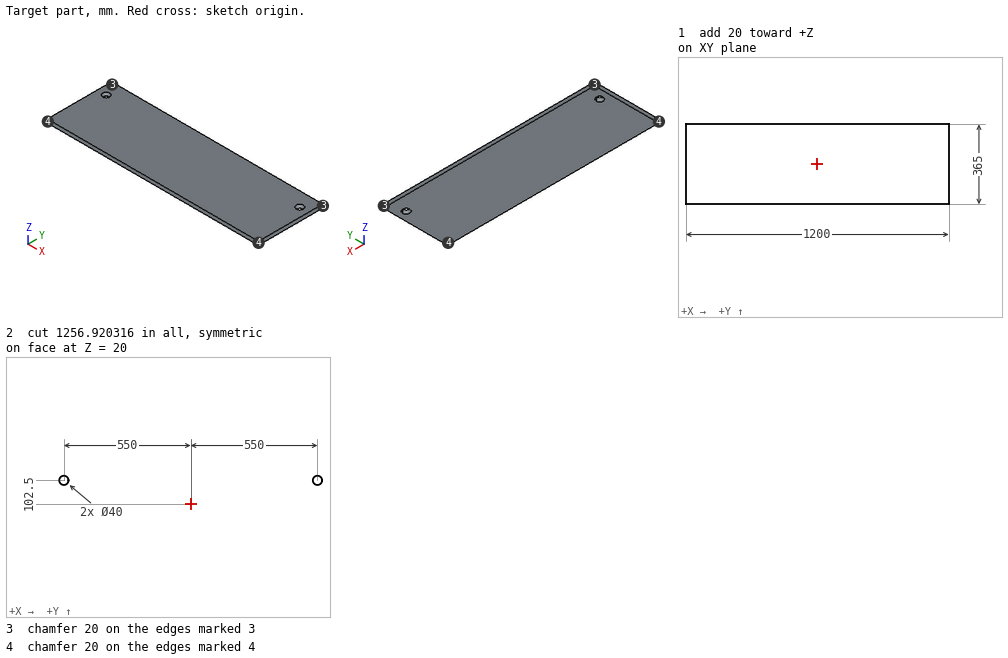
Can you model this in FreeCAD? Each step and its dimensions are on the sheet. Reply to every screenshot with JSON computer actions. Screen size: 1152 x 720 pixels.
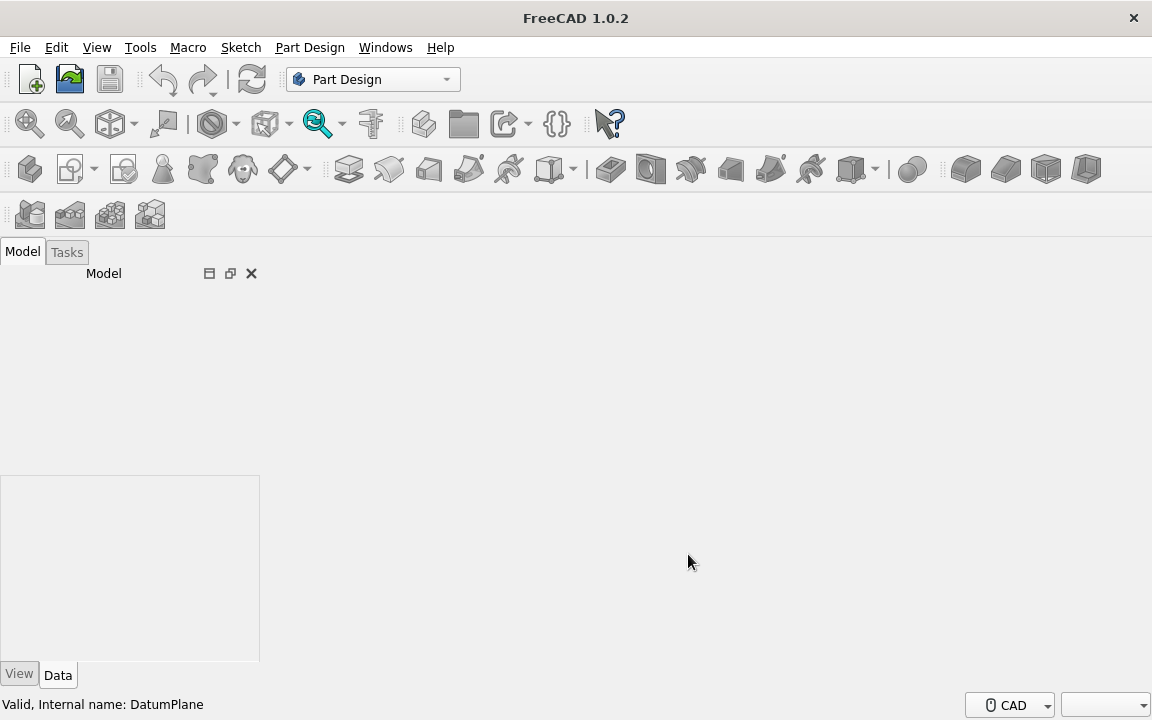
{"action": "left_click", "coordinate": [30, 80]}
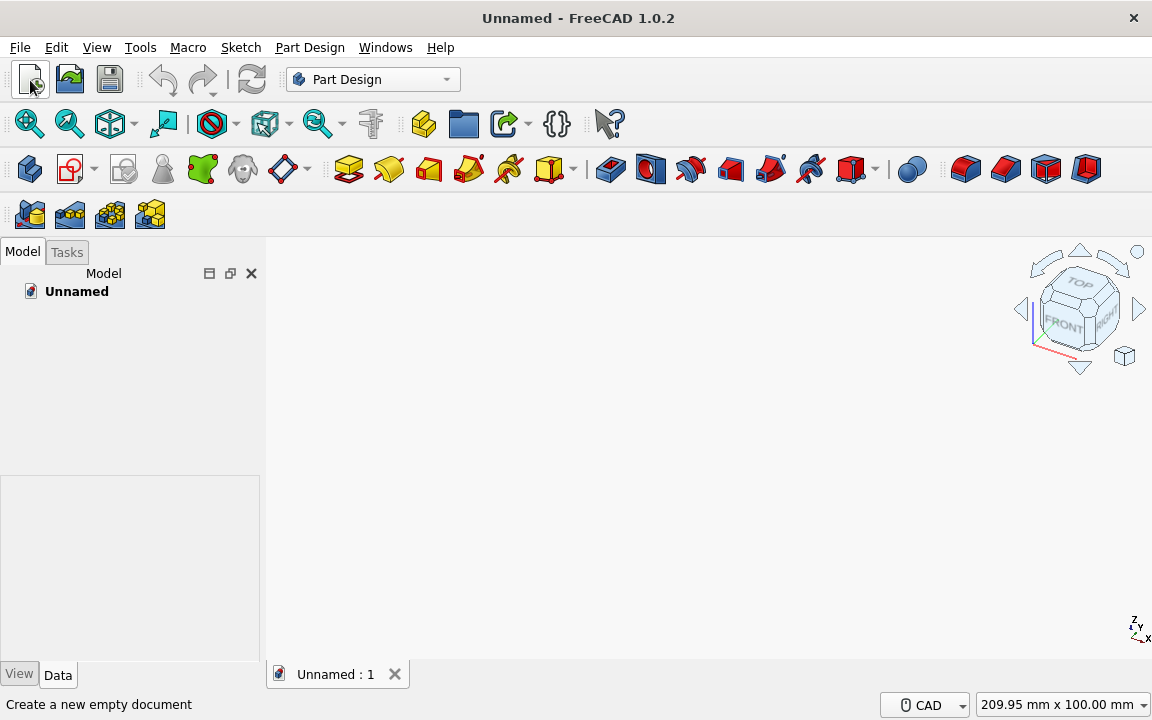
{"action": "left_click", "coordinate": [70, 170]}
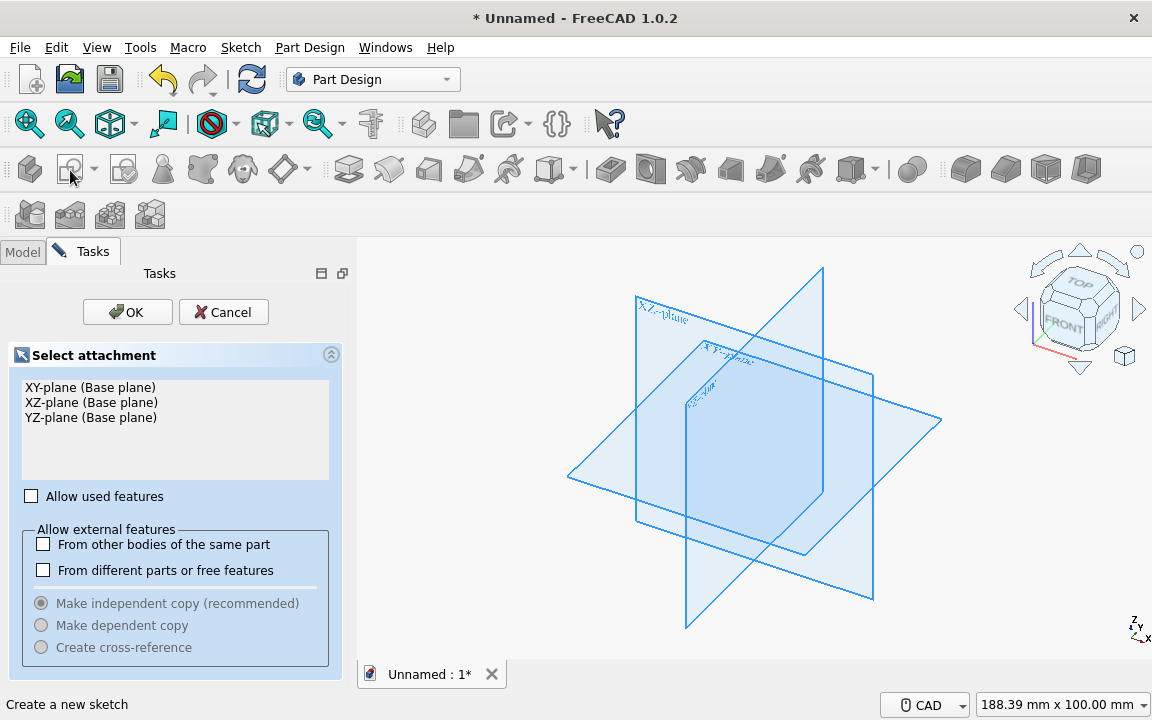
{"action": "left_click", "coordinate": [82, 388]}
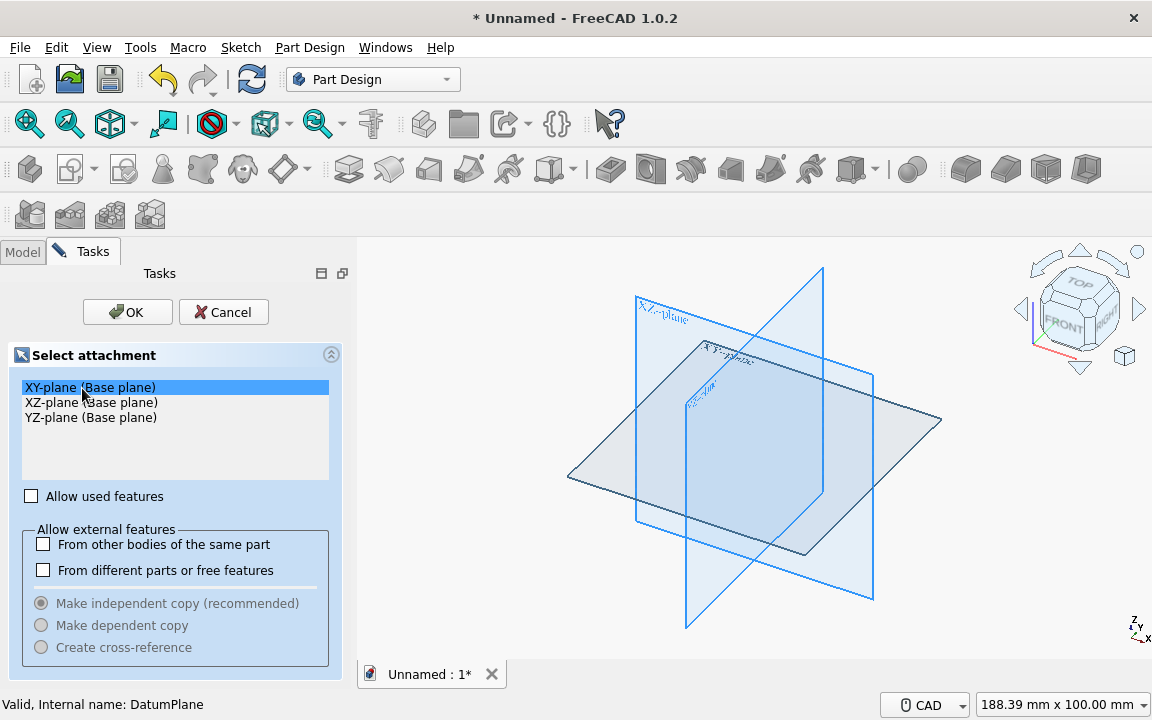
{"action": "left_click", "coordinate": [128, 312]}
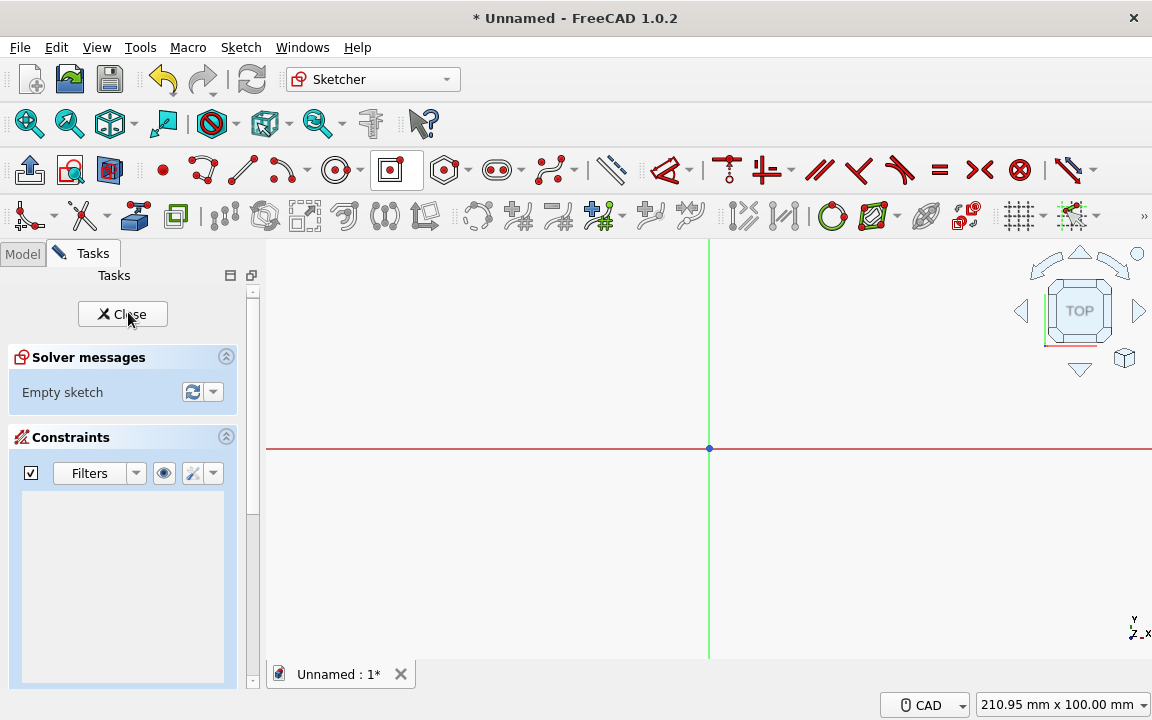
{"action": "scroll", "coordinate": [634, 449], "scroll_direction": "down", "scroll_amount": 12}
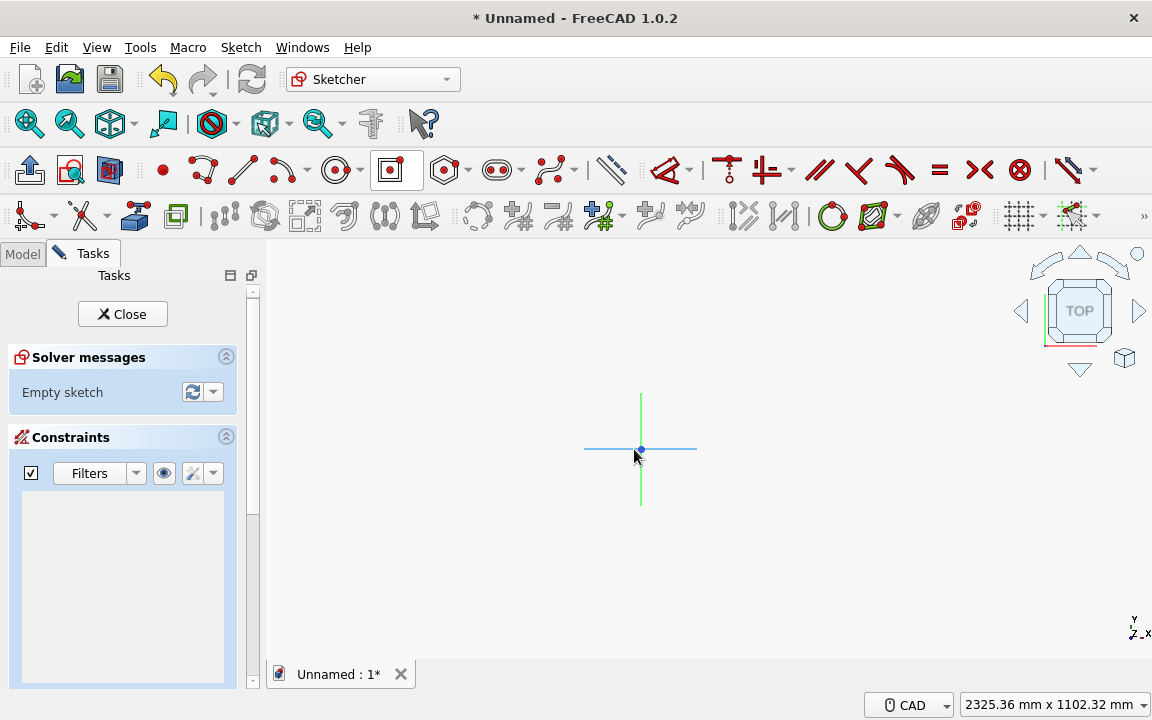
{"action": "key", "text": "g v"}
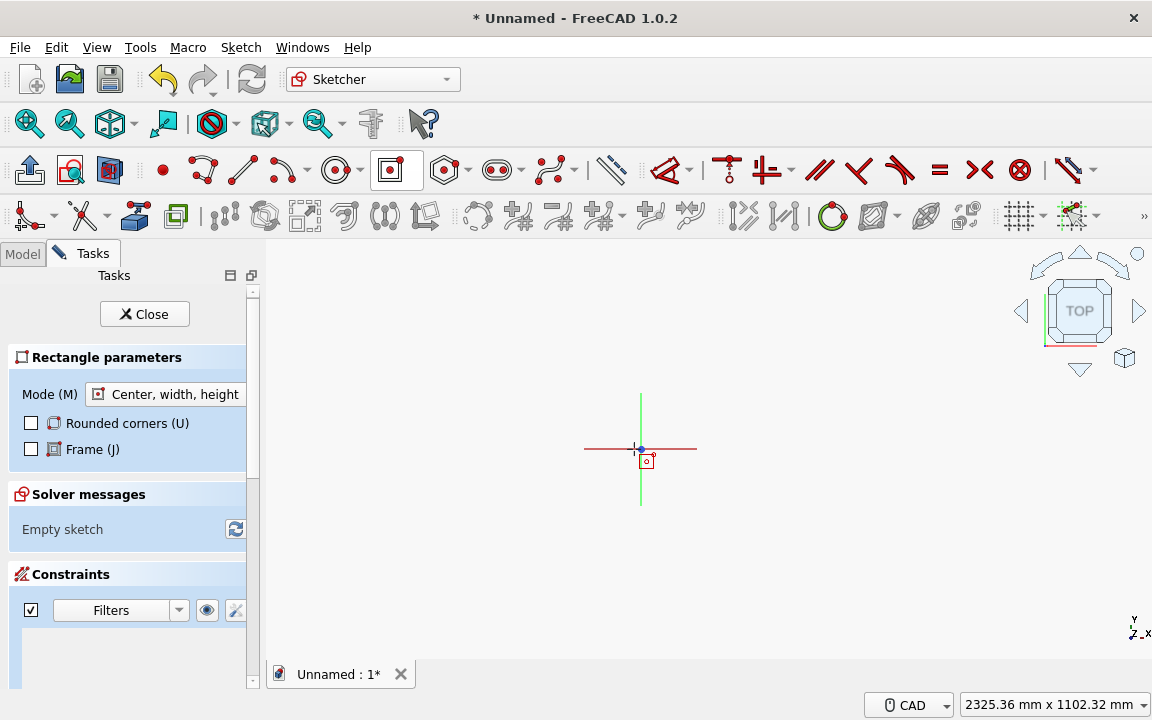
{"action": "left_click", "coordinate": [641, 449]}
{"action": "mouse_move", "coordinate": [870, 380]}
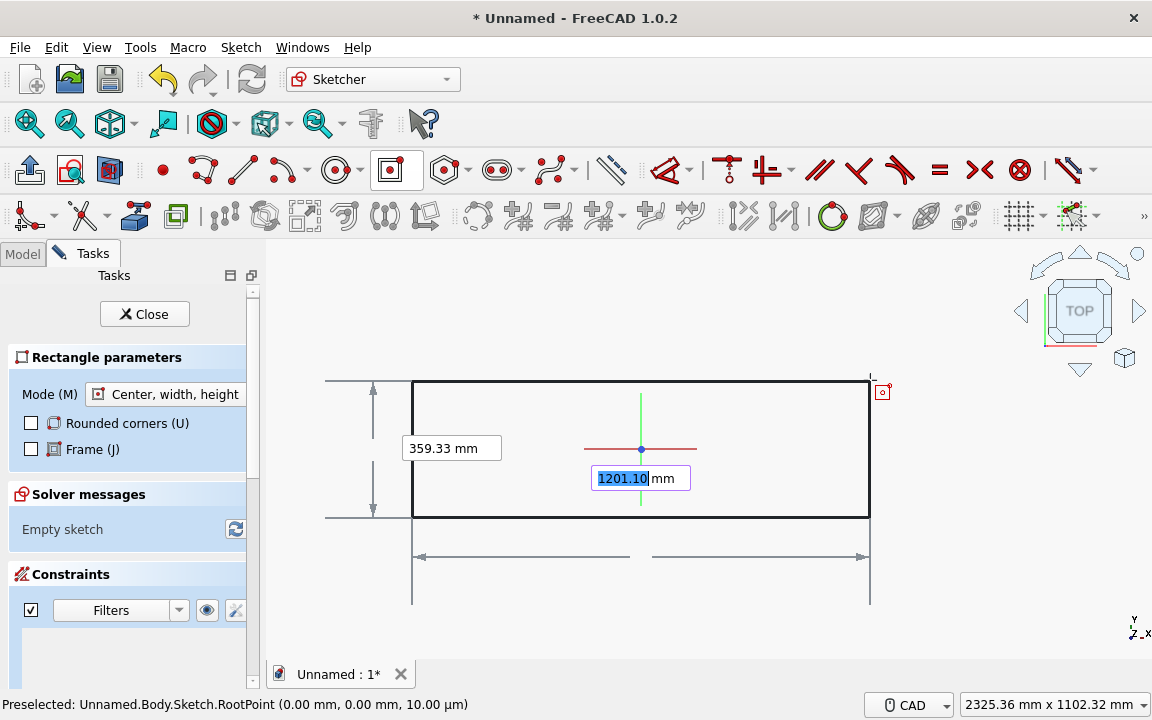
{"action": "type", "text": "1200"}
{"action": "key", "text": "Tab"}
{"action": "type", "text": "365"}
{"action": "key", "text": "Return"}
{"action": "key", "text": "Escape"}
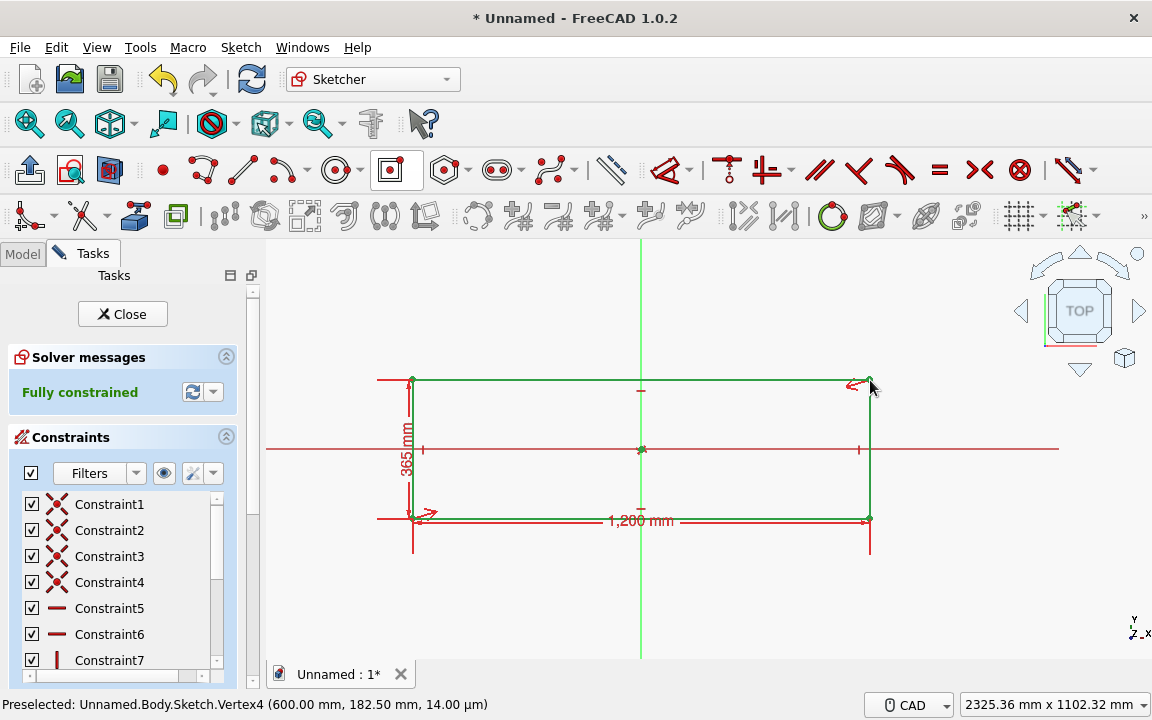
{"action": "left_click", "coordinate": [123, 314]}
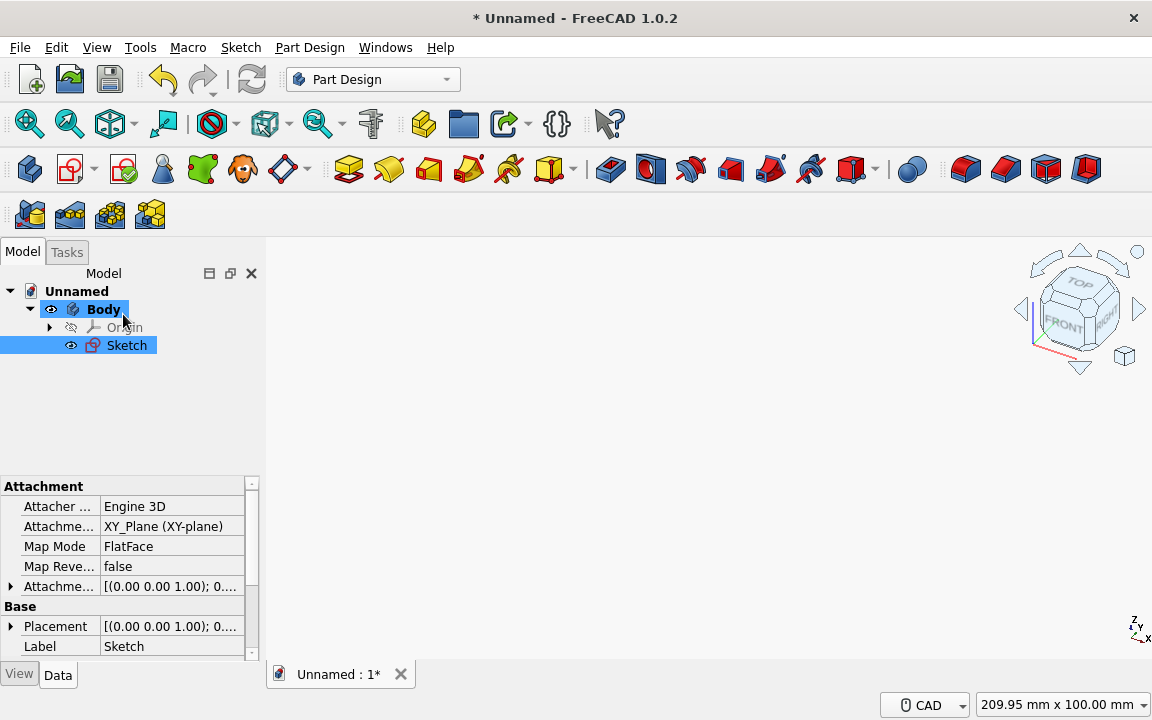
{"action": "left_click", "coordinate": [350, 170]}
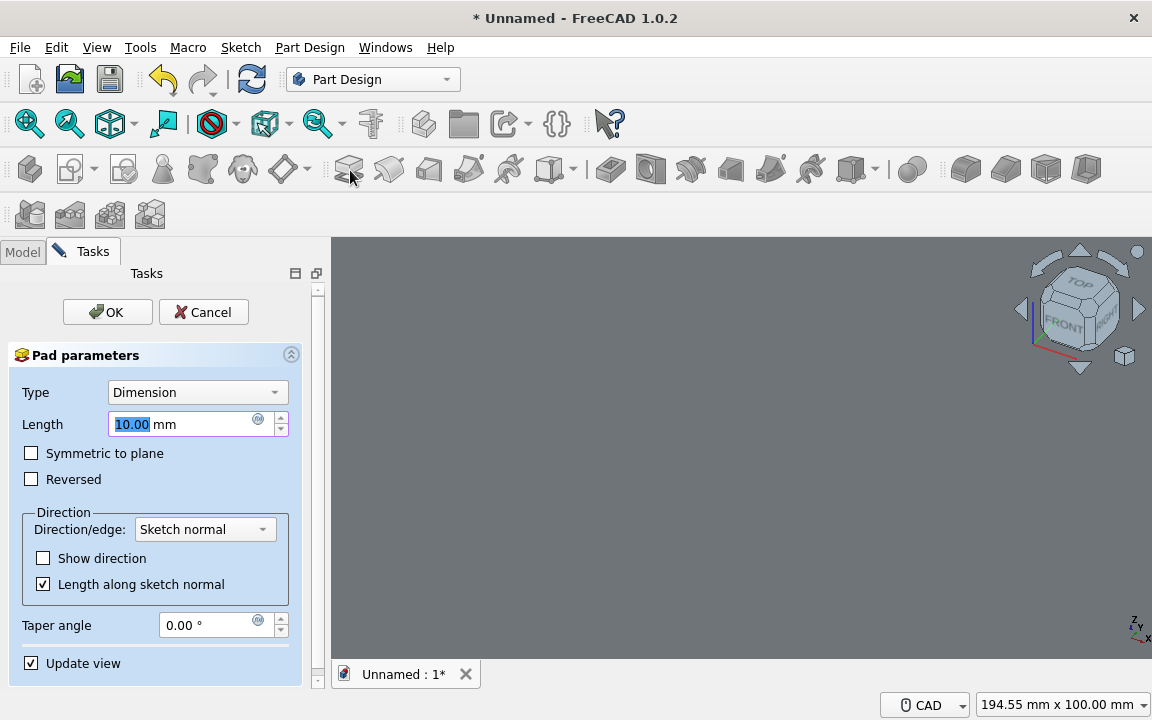
{"action": "type", "text": "20"}
{"action": "key", "text": "Tab"}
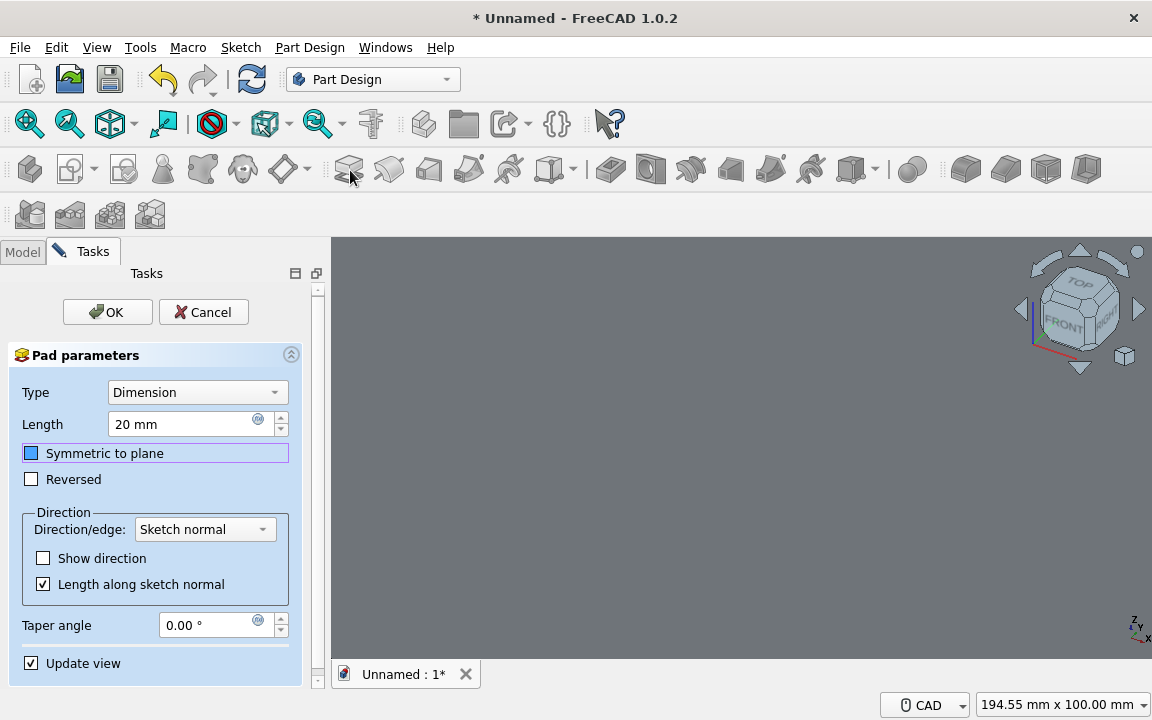
{"action": "left_click", "coordinate": [108, 312]}